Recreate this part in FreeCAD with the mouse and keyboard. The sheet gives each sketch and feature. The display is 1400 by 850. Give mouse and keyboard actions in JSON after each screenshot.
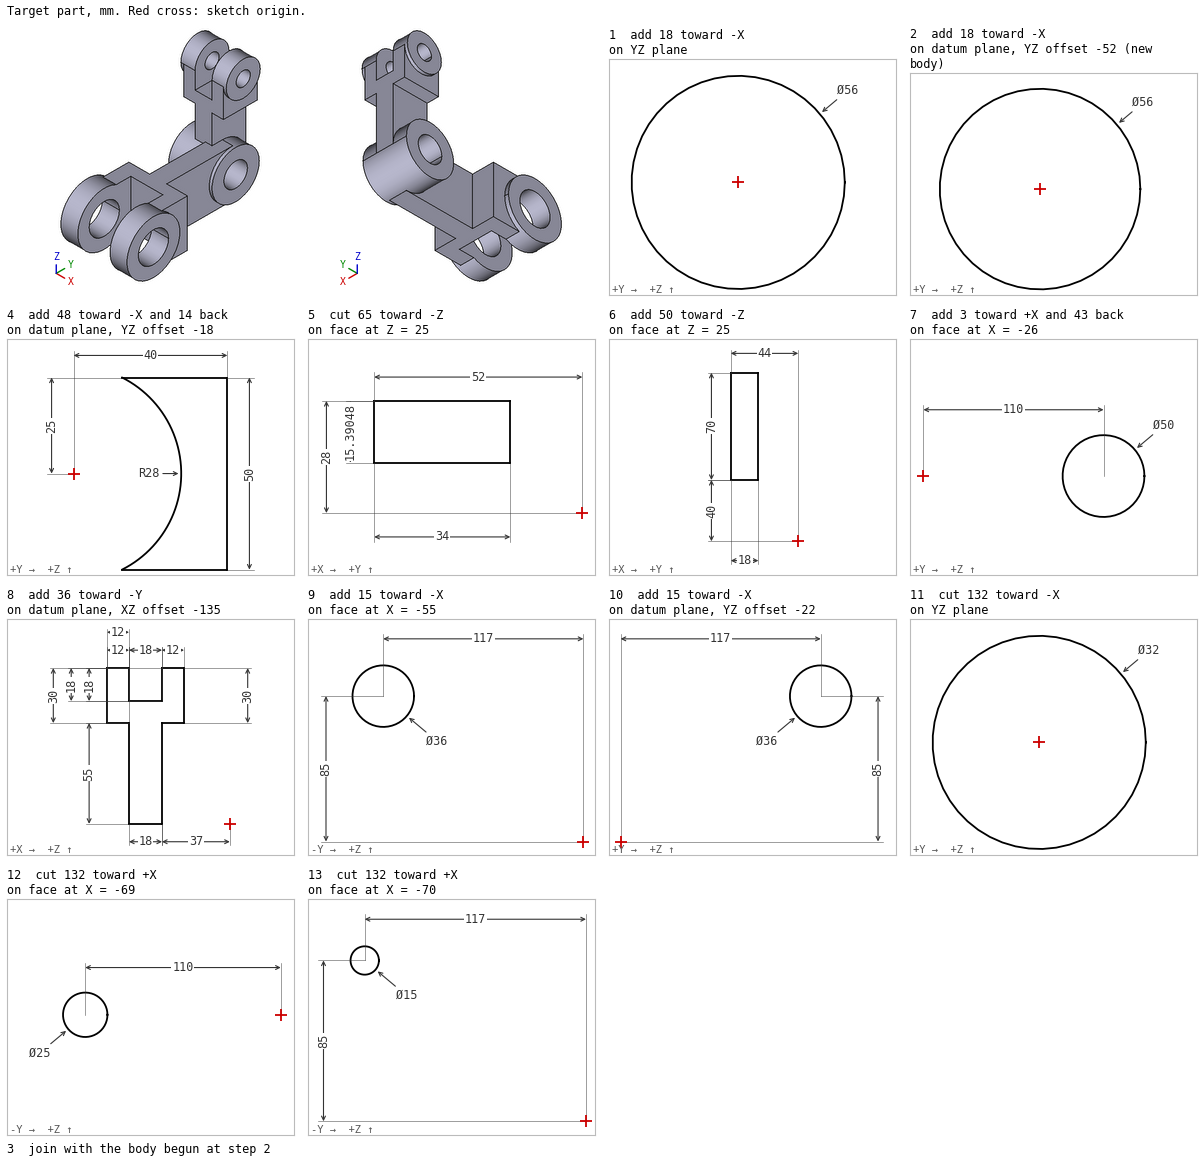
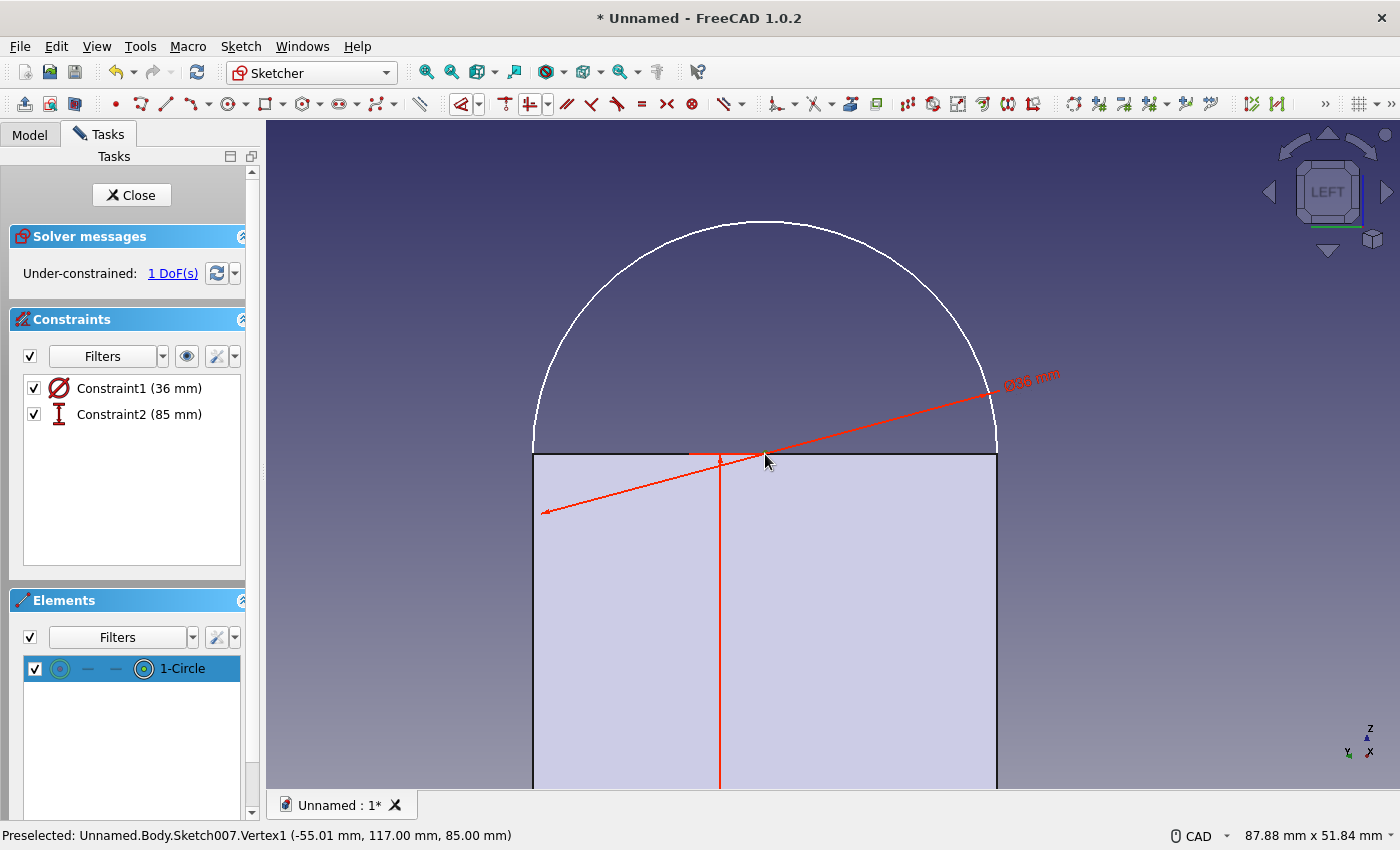
{"action": "left_click", "coordinate": [478, 104]}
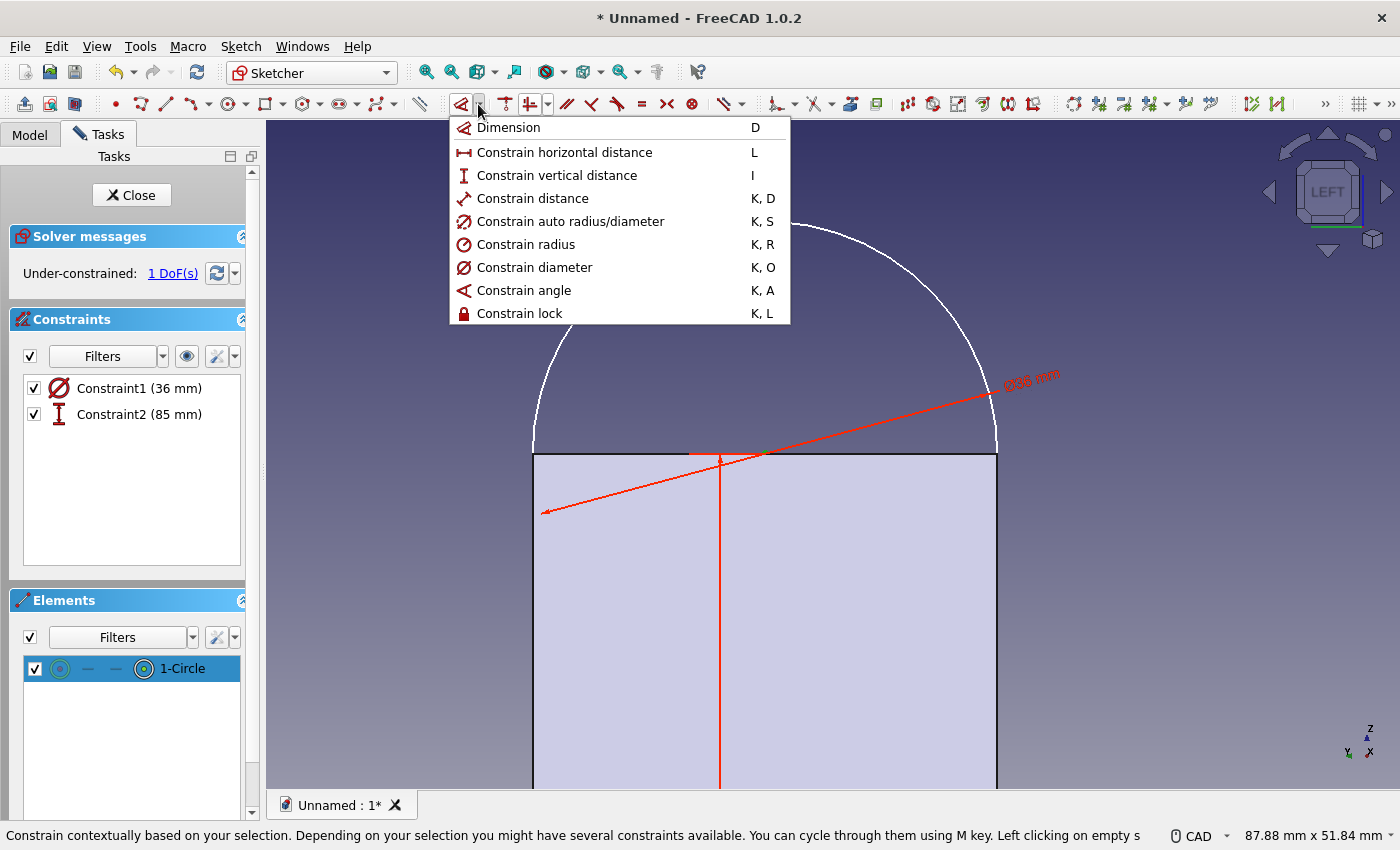
{"action": "left_click", "coordinate": [620, 152]}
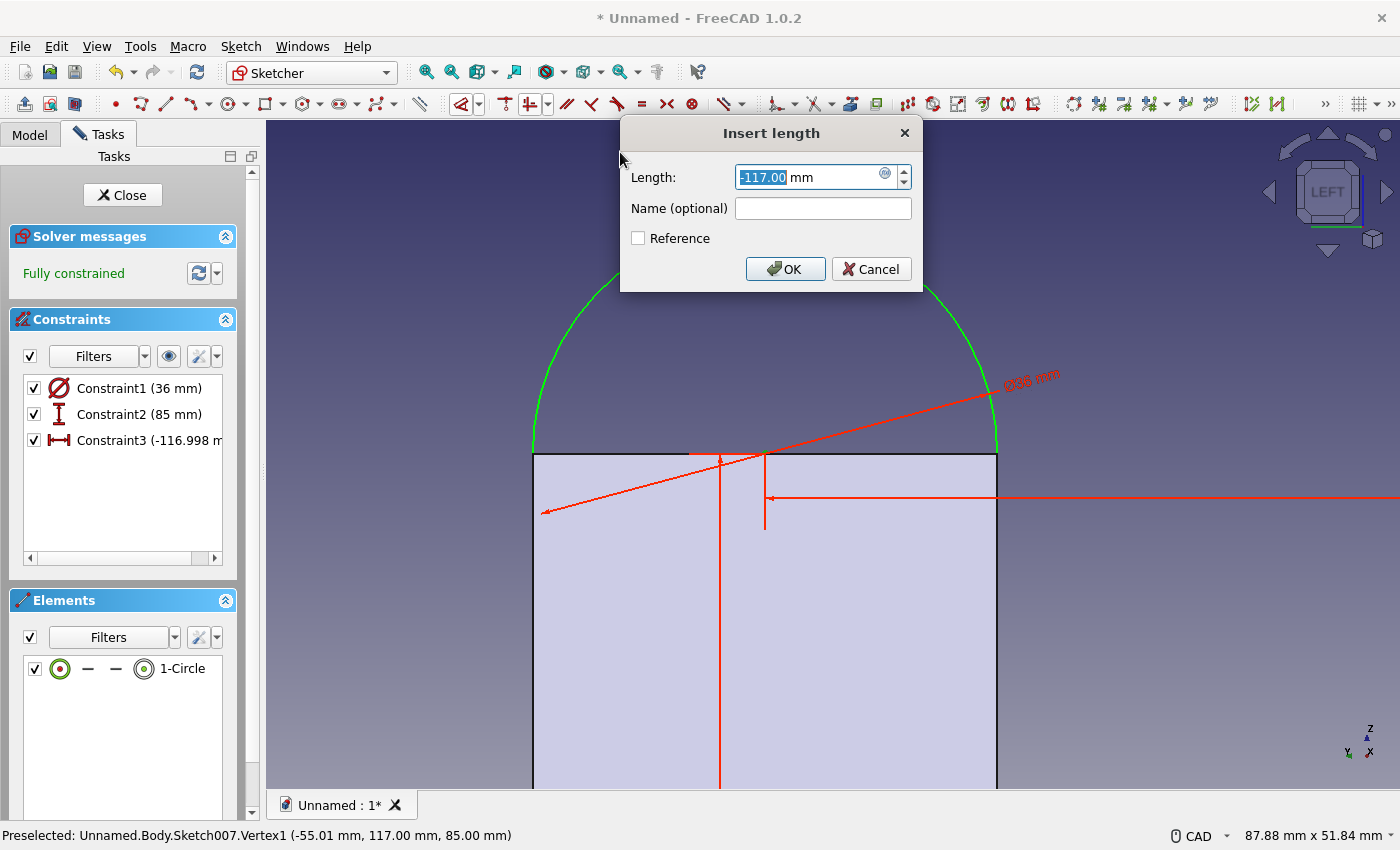
{"action": "type", "text": "-117"}
{"action": "key", "text": "Return"}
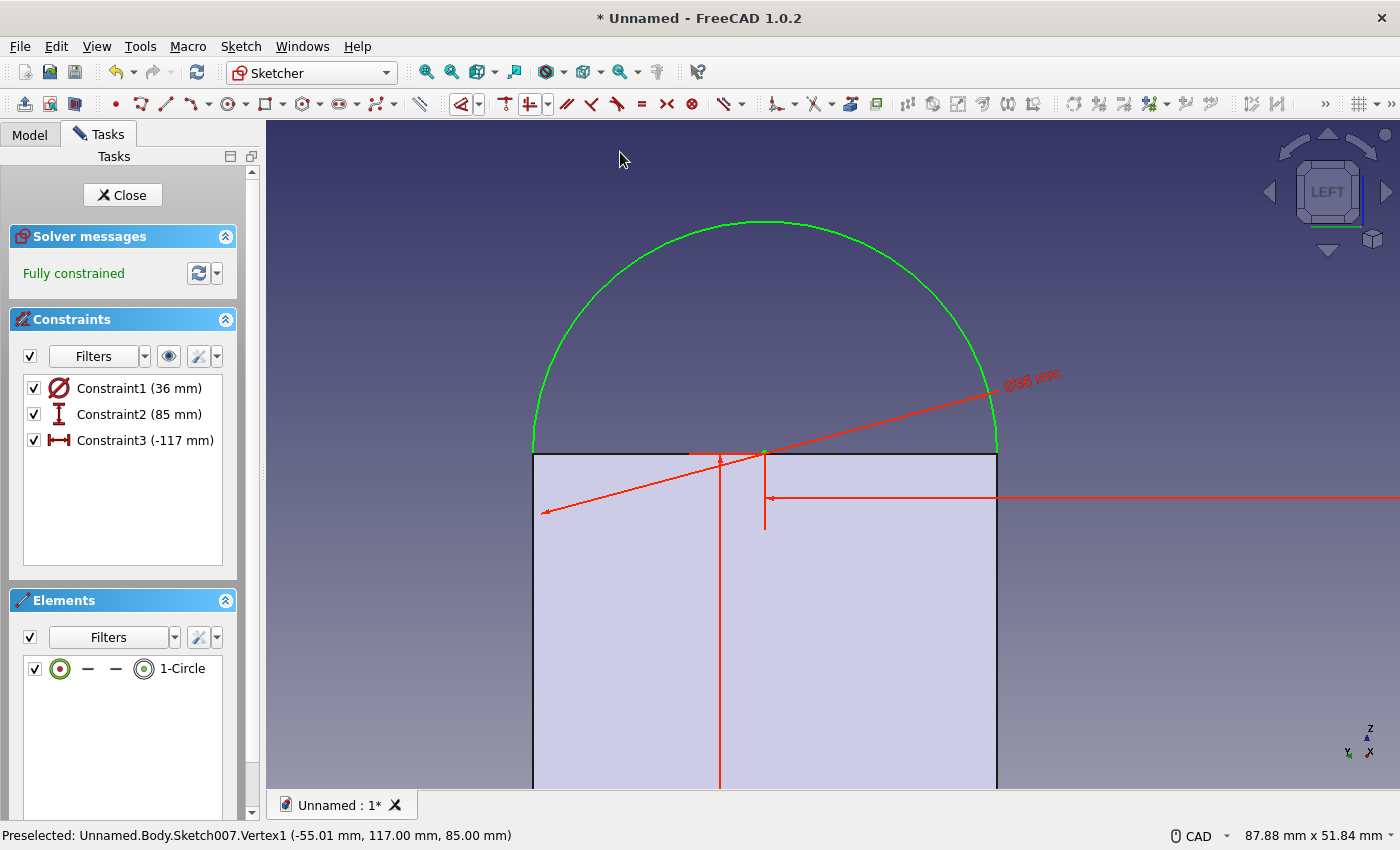
{"action": "left_click", "coordinate": [123, 195]}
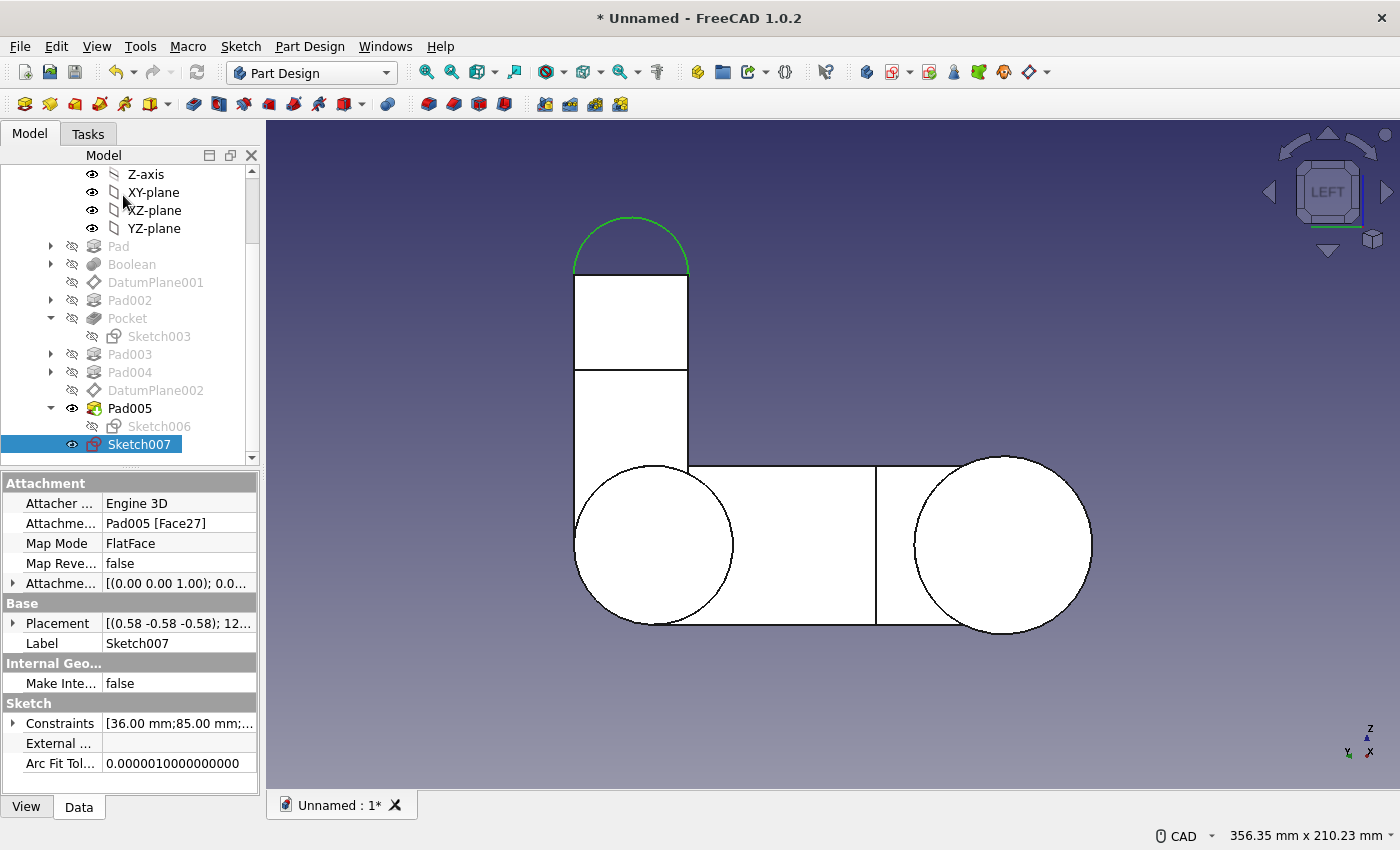
{"action": "left_click", "coordinate": [25, 104]}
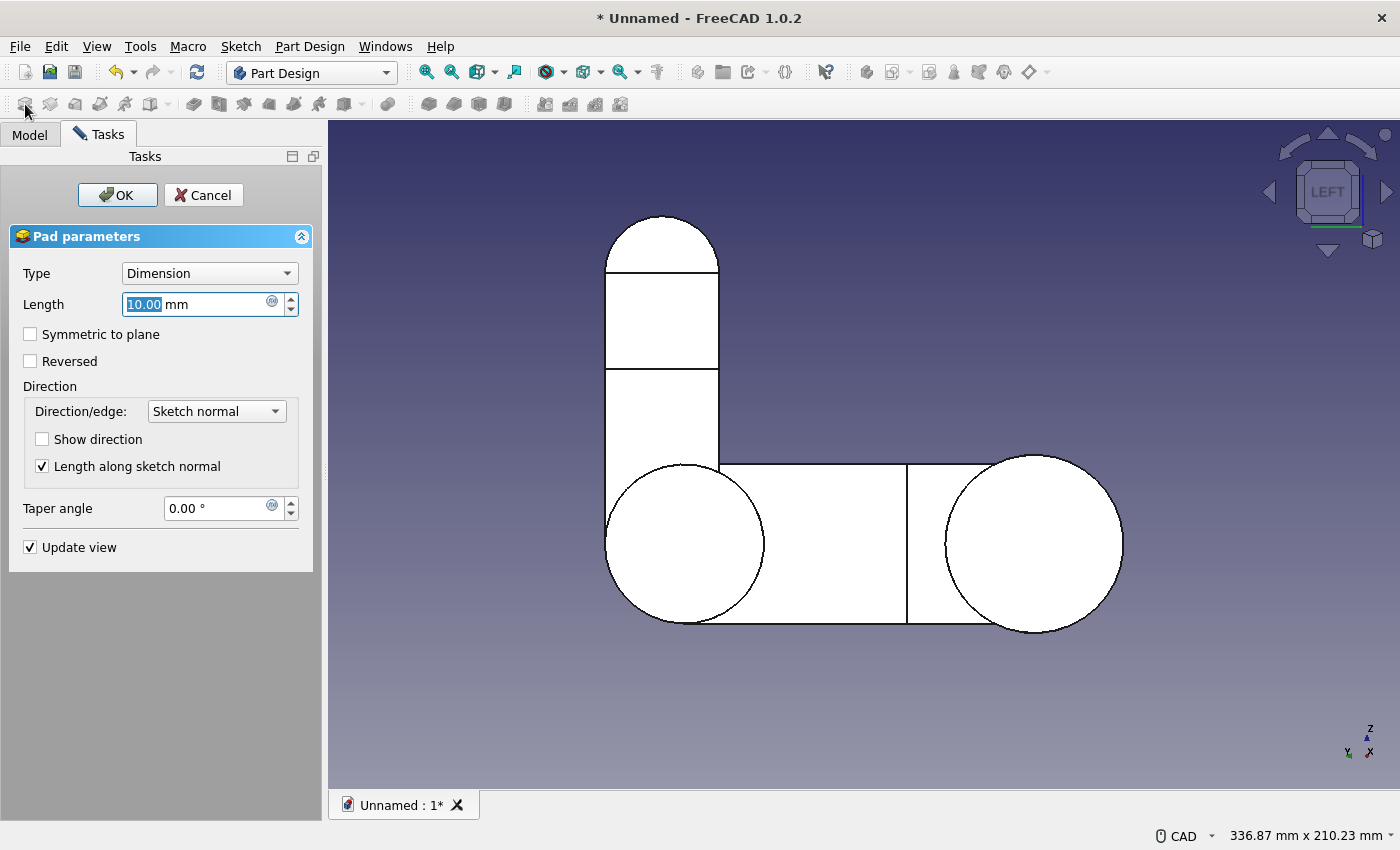
{"action": "type", "text": "15"}
{"action": "key", "text": "Tab"}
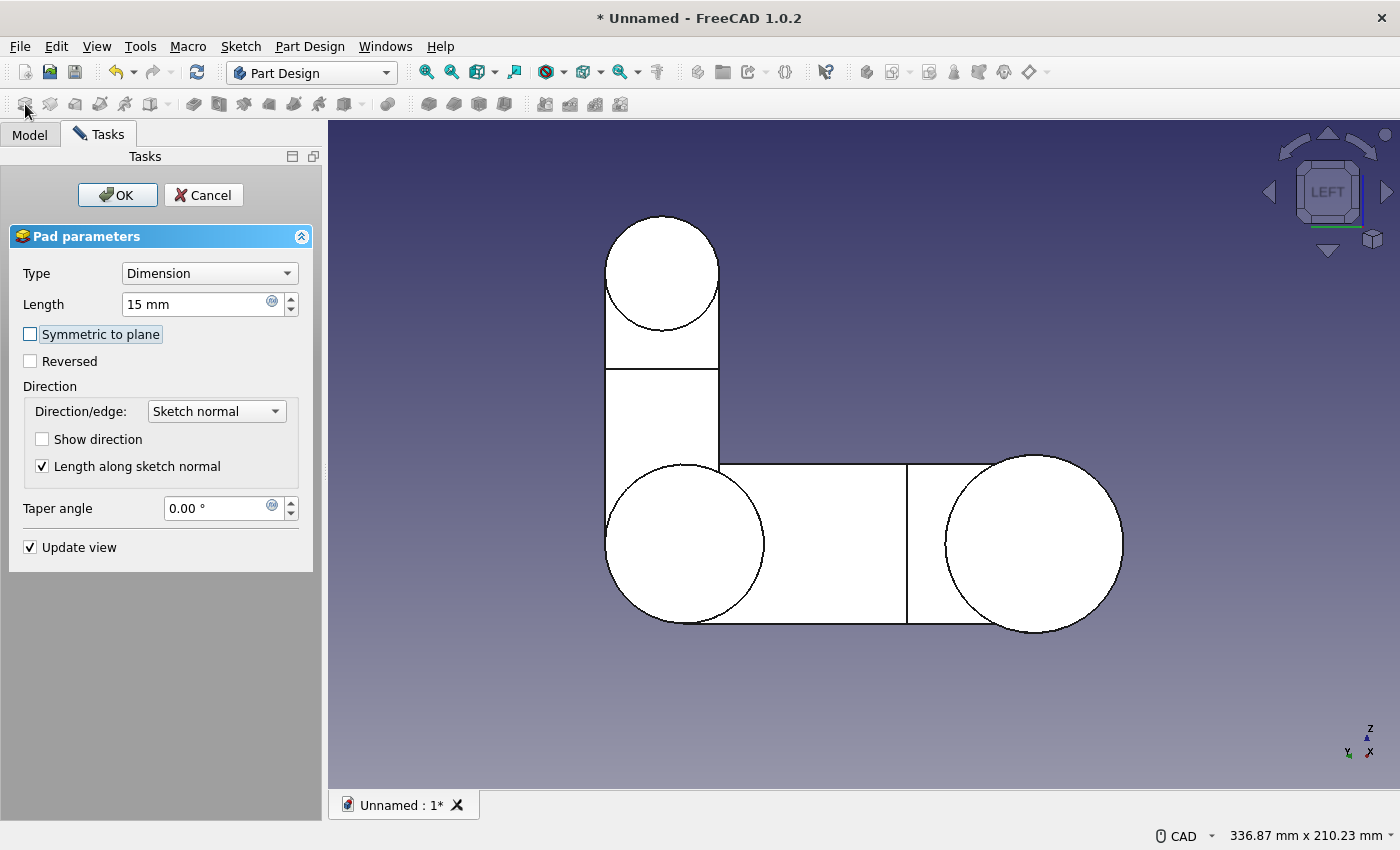
{"action": "left_click", "coordinate": [118, 195]}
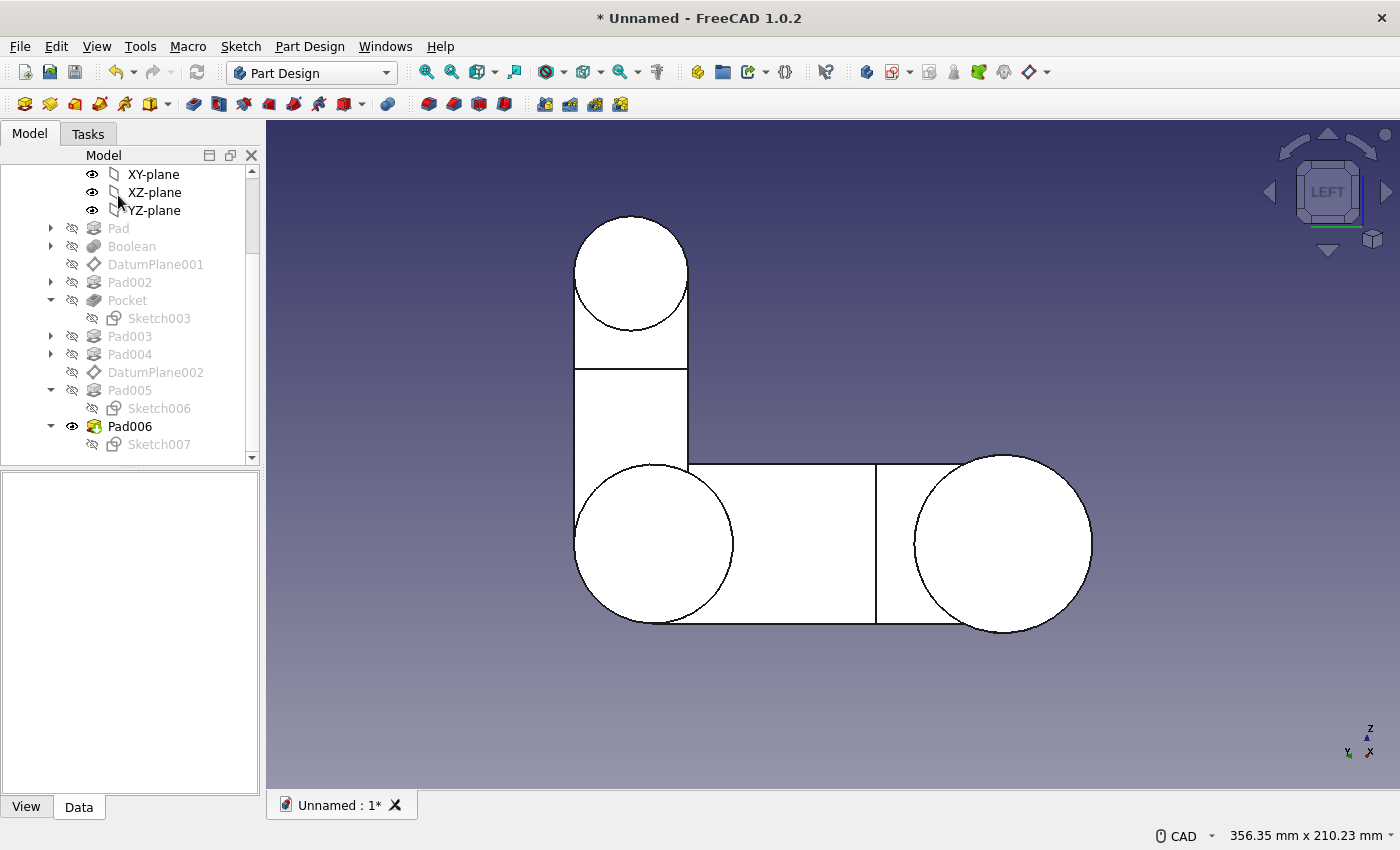
{"action": "scroll", "coordinate": [161, 314], "scroll_direction": "down", "scroll_amount": 3}